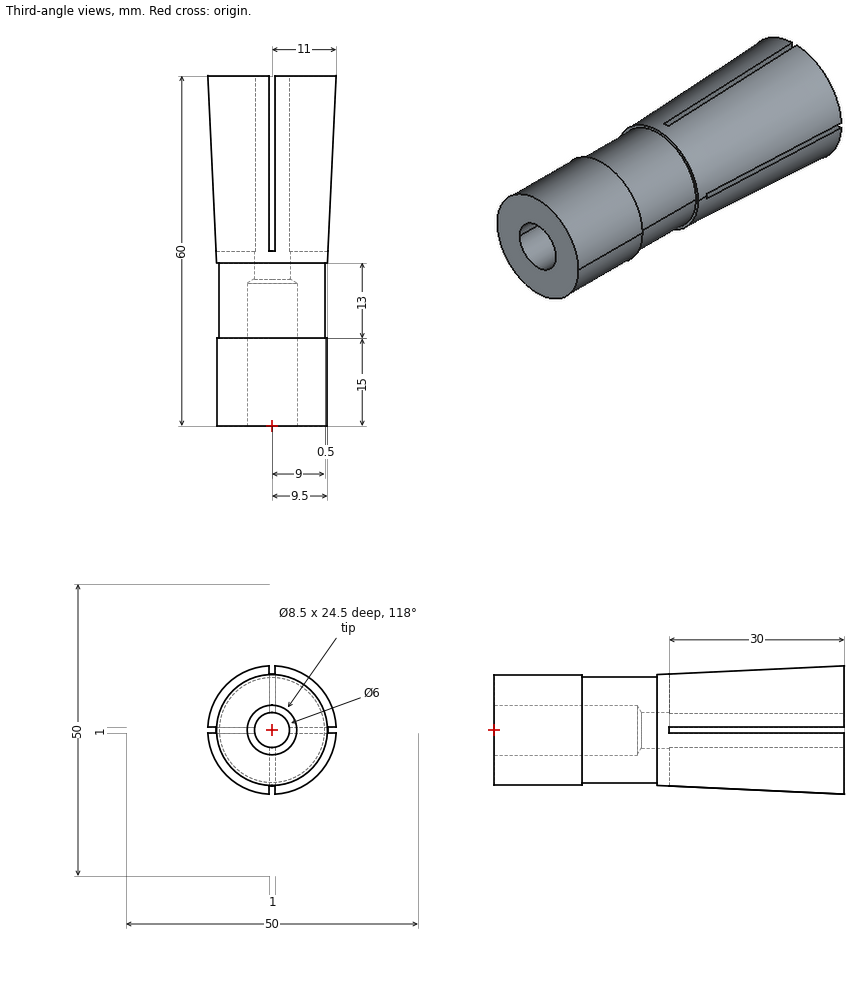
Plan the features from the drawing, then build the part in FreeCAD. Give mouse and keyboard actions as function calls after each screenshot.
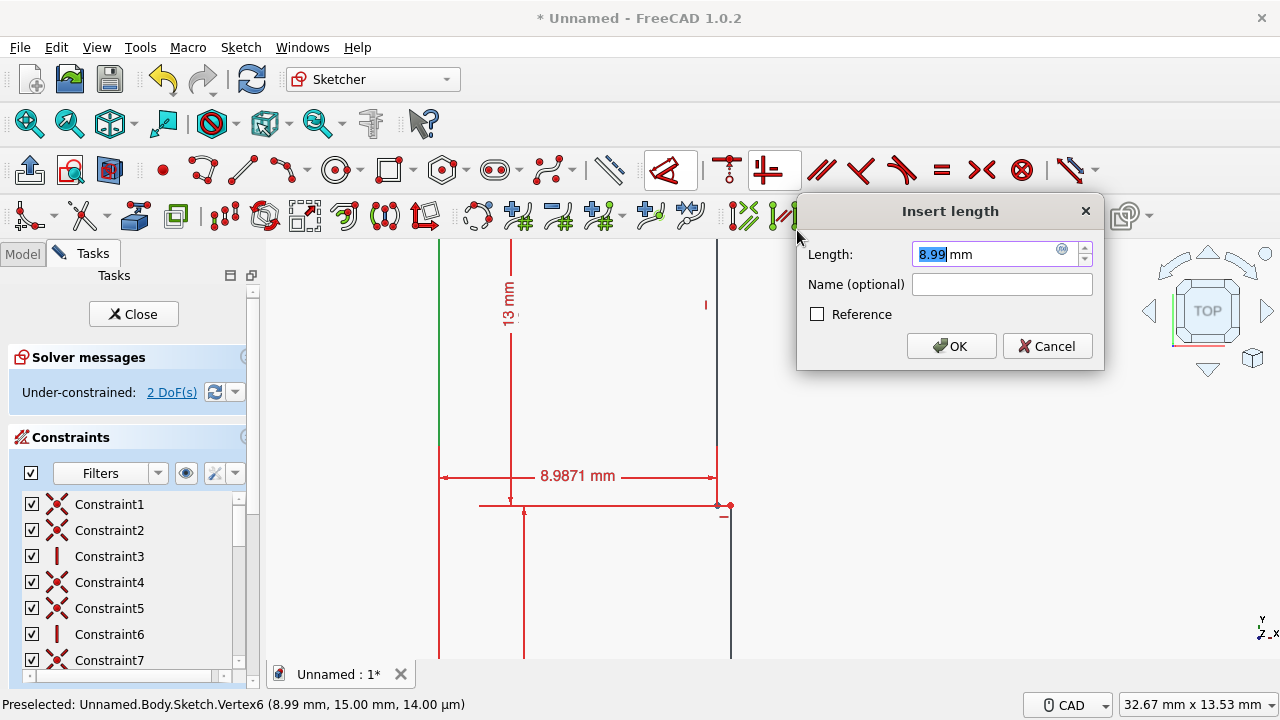
text(9)
key(Return)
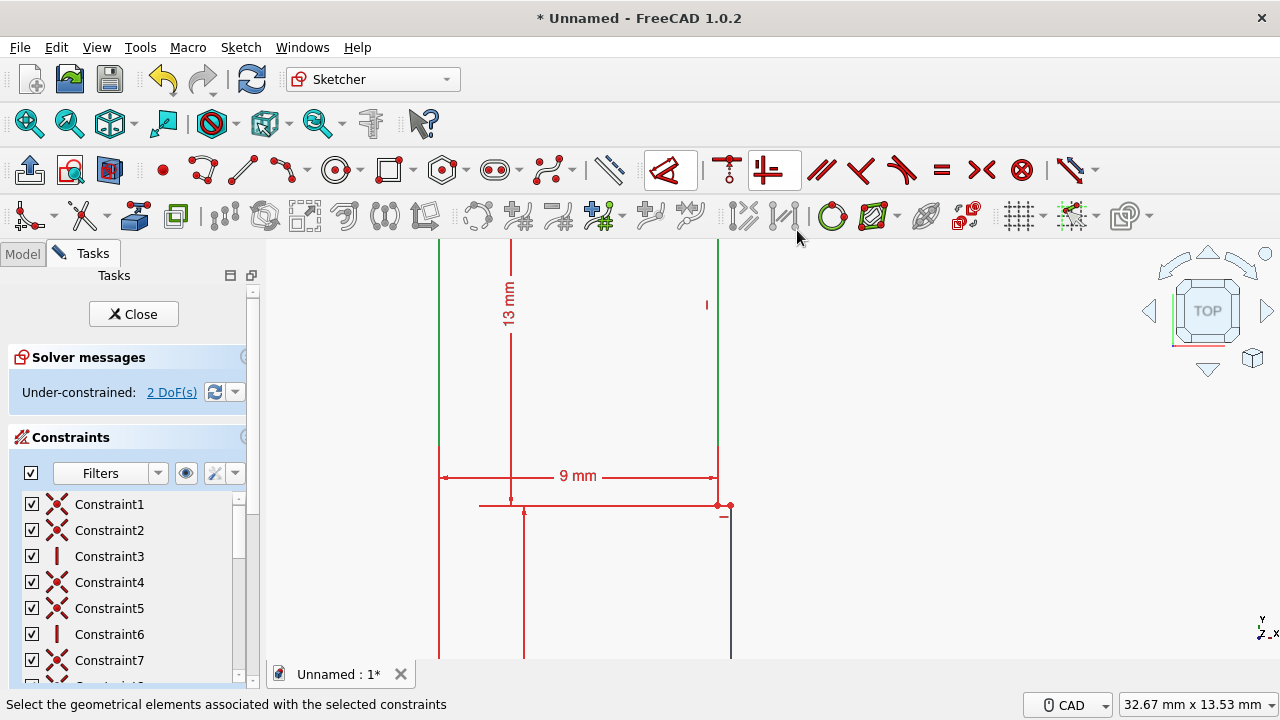
scroll(719, 513, down, 10)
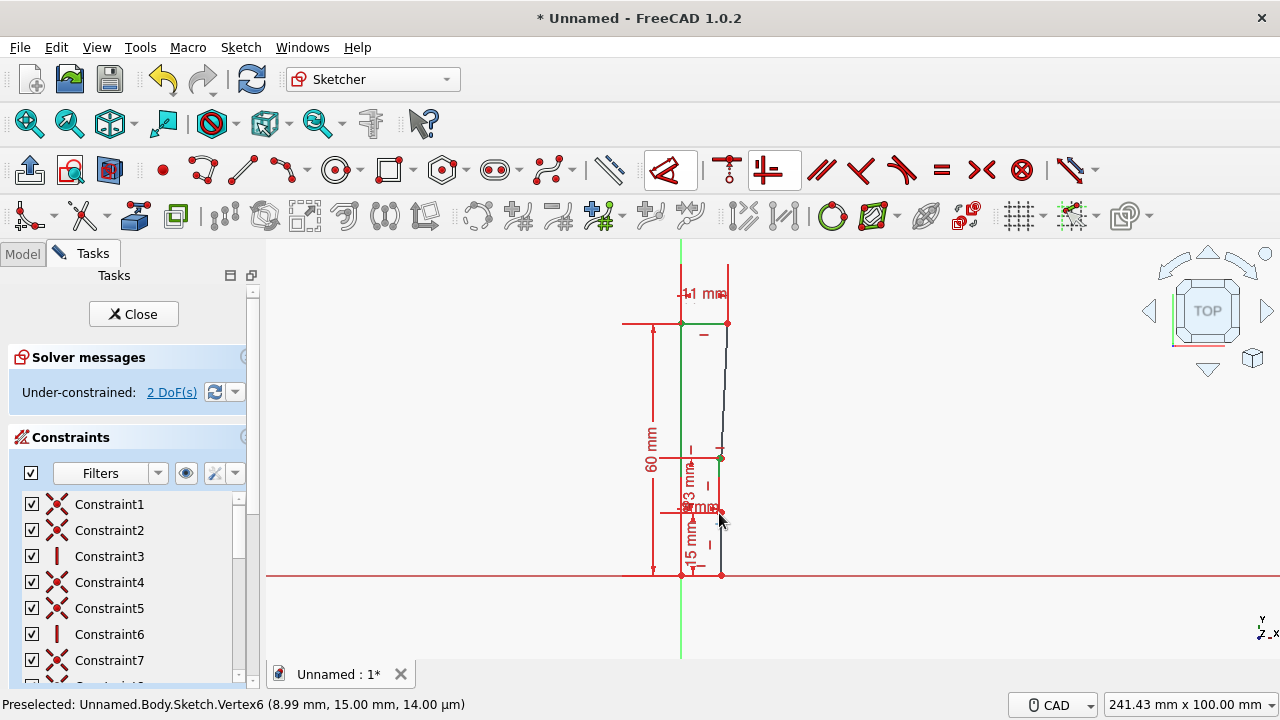
click(693, 576)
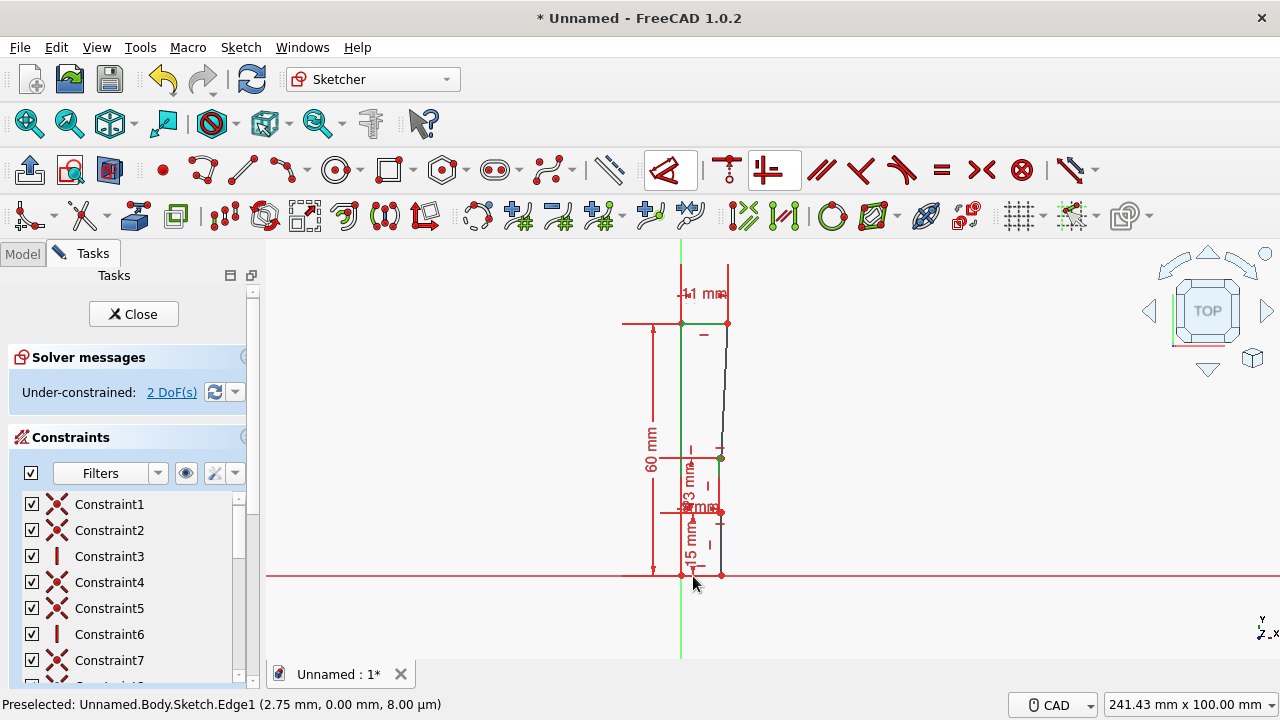
key(l)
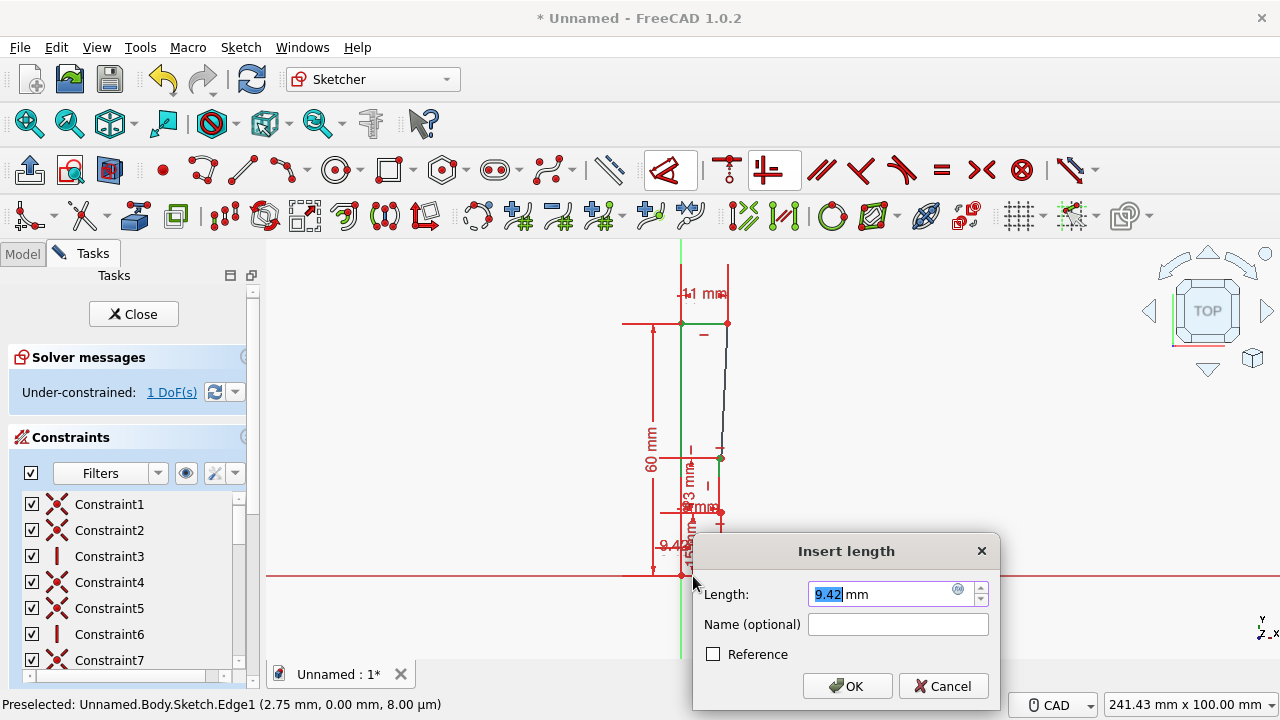
text(9.5)
key(Return)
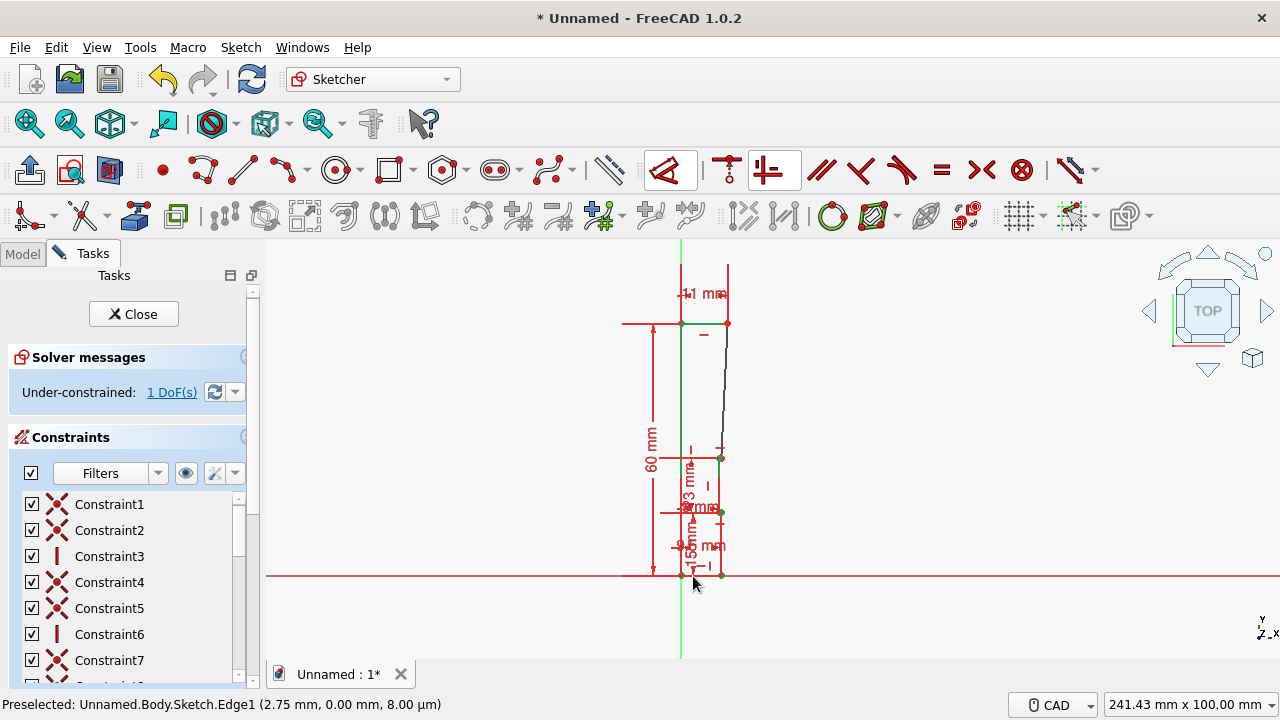
scroll(720, 458, up, 15)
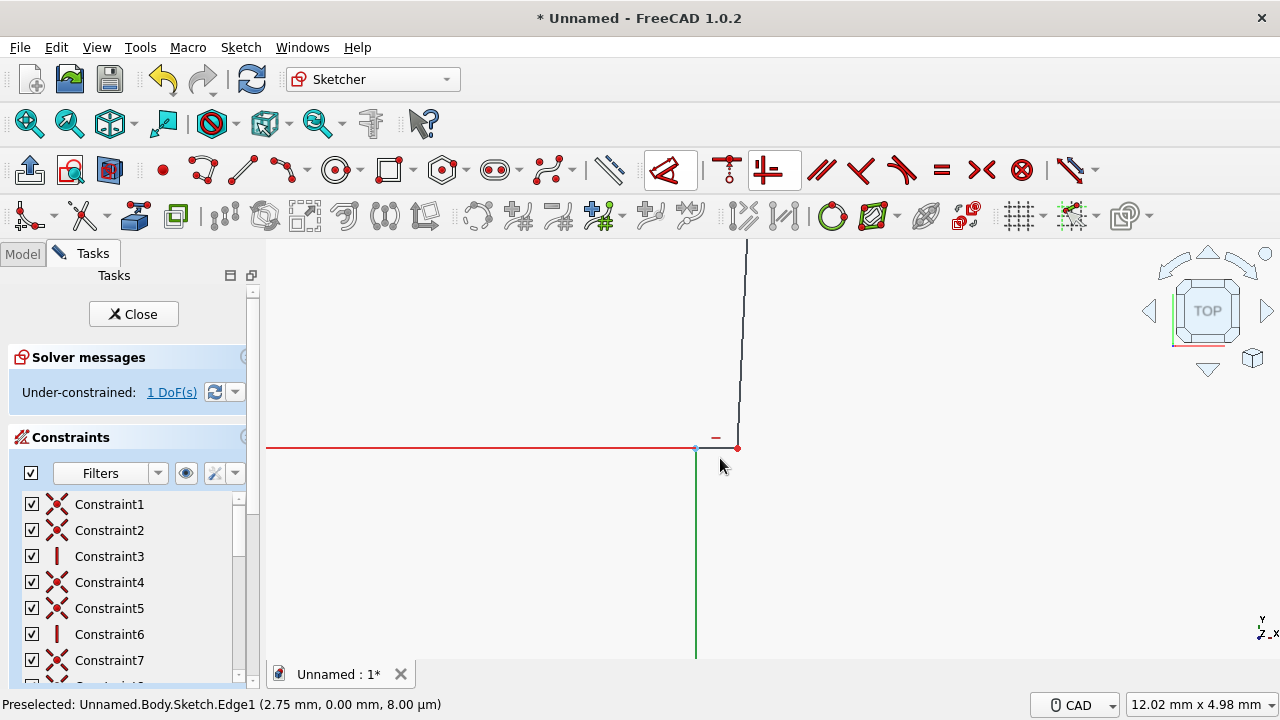
click(717, 448)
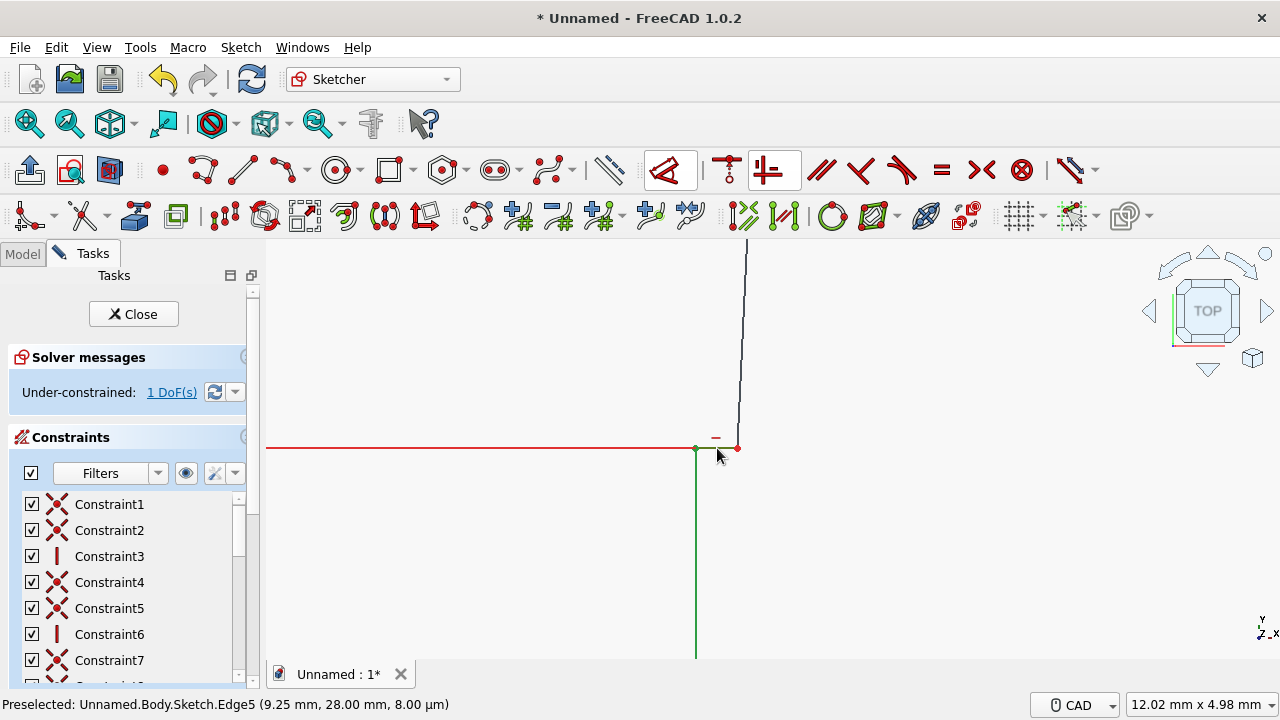
click(692, 170)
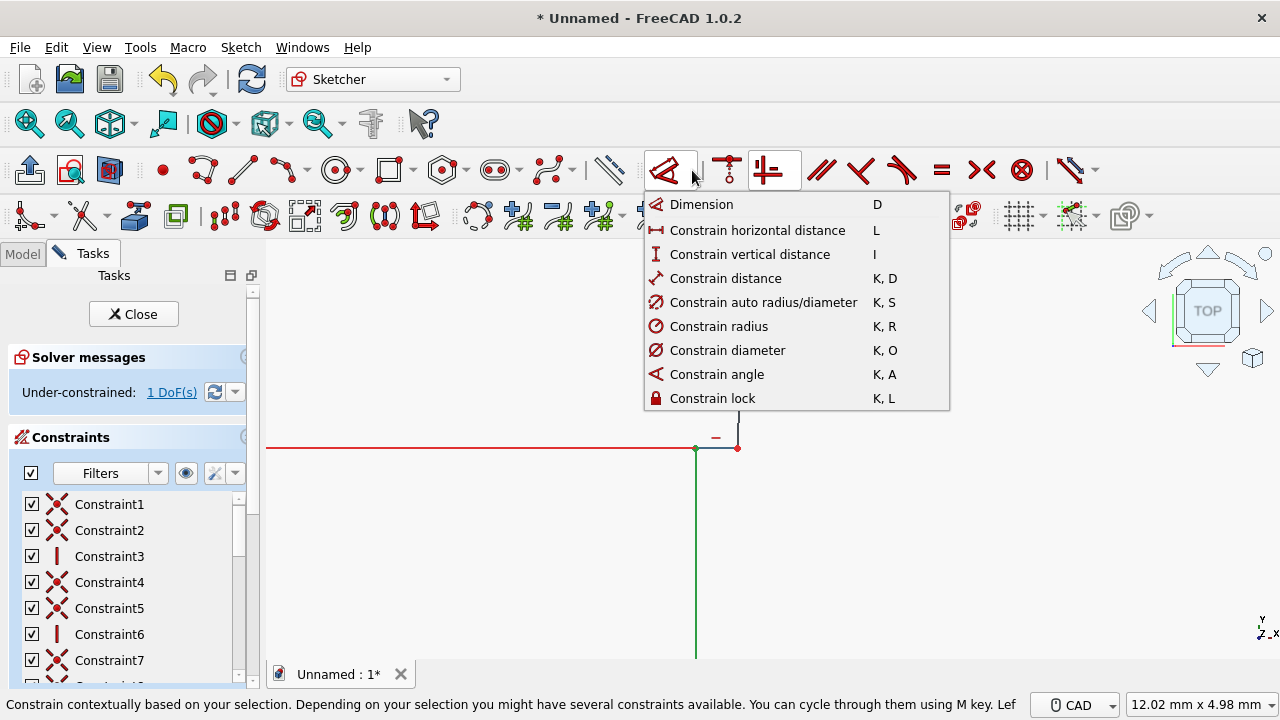
click(797, 230)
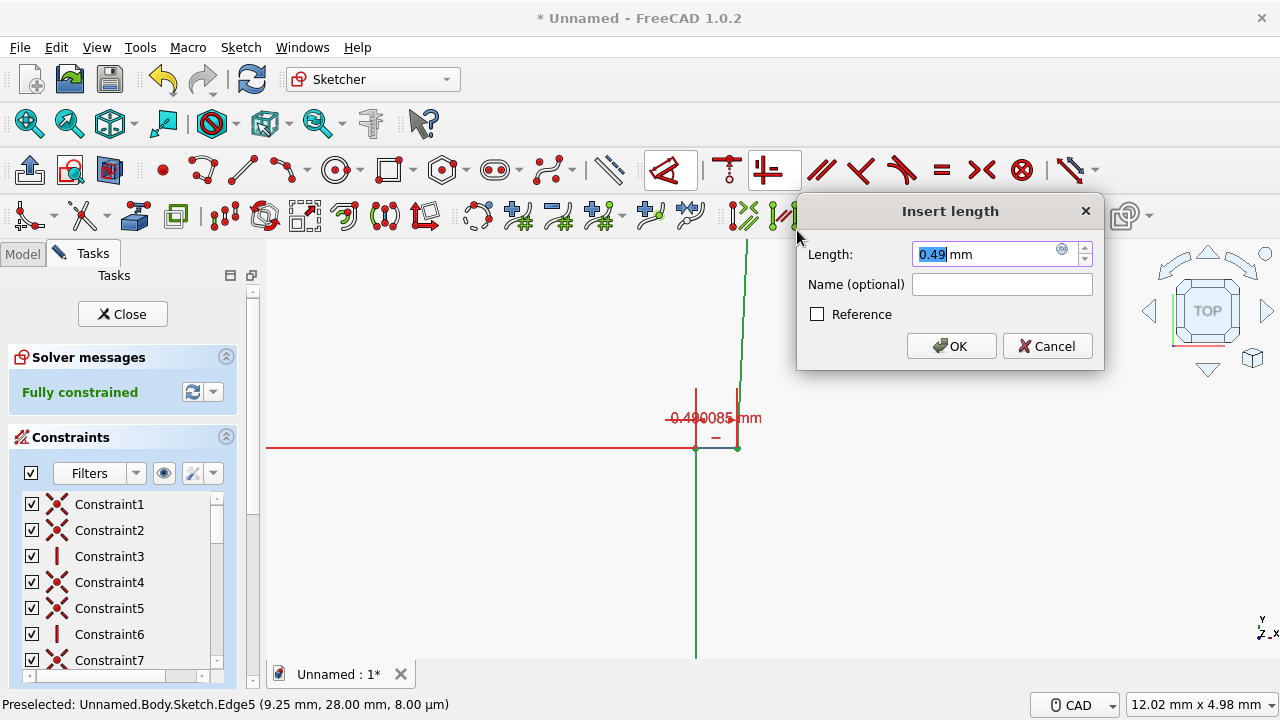
text(0.5)
key(Return)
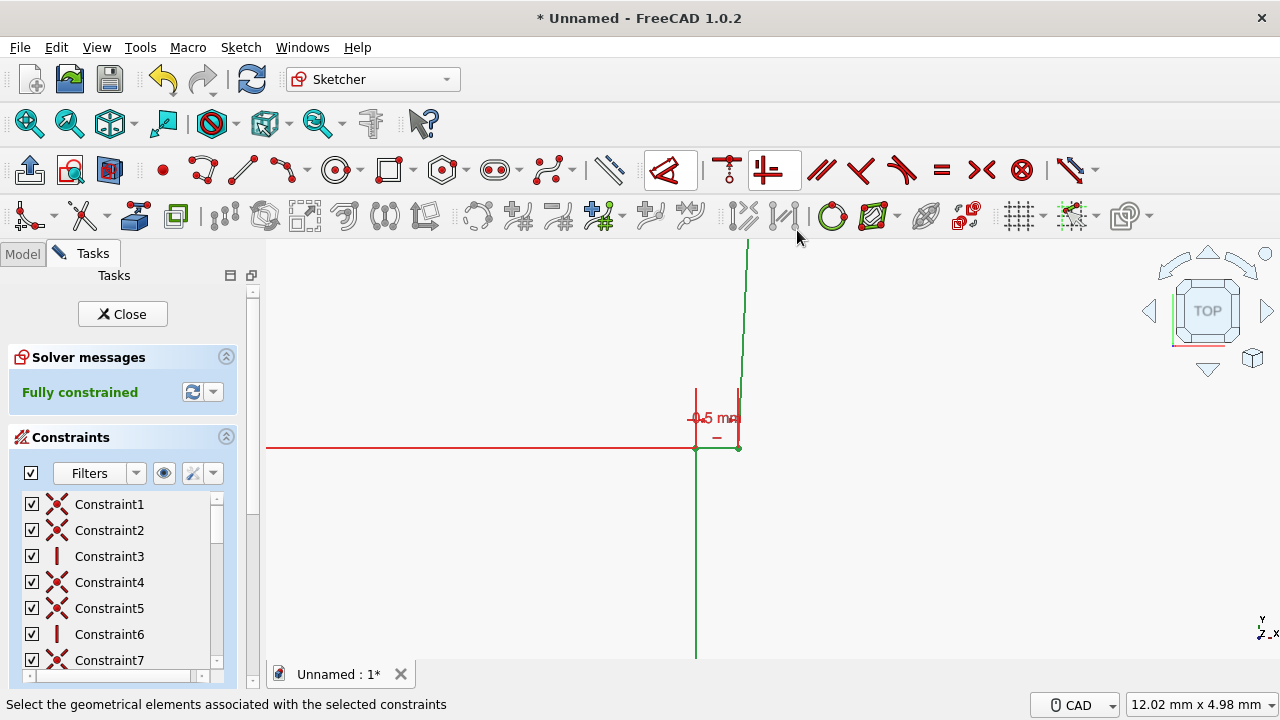
click(123, 314)